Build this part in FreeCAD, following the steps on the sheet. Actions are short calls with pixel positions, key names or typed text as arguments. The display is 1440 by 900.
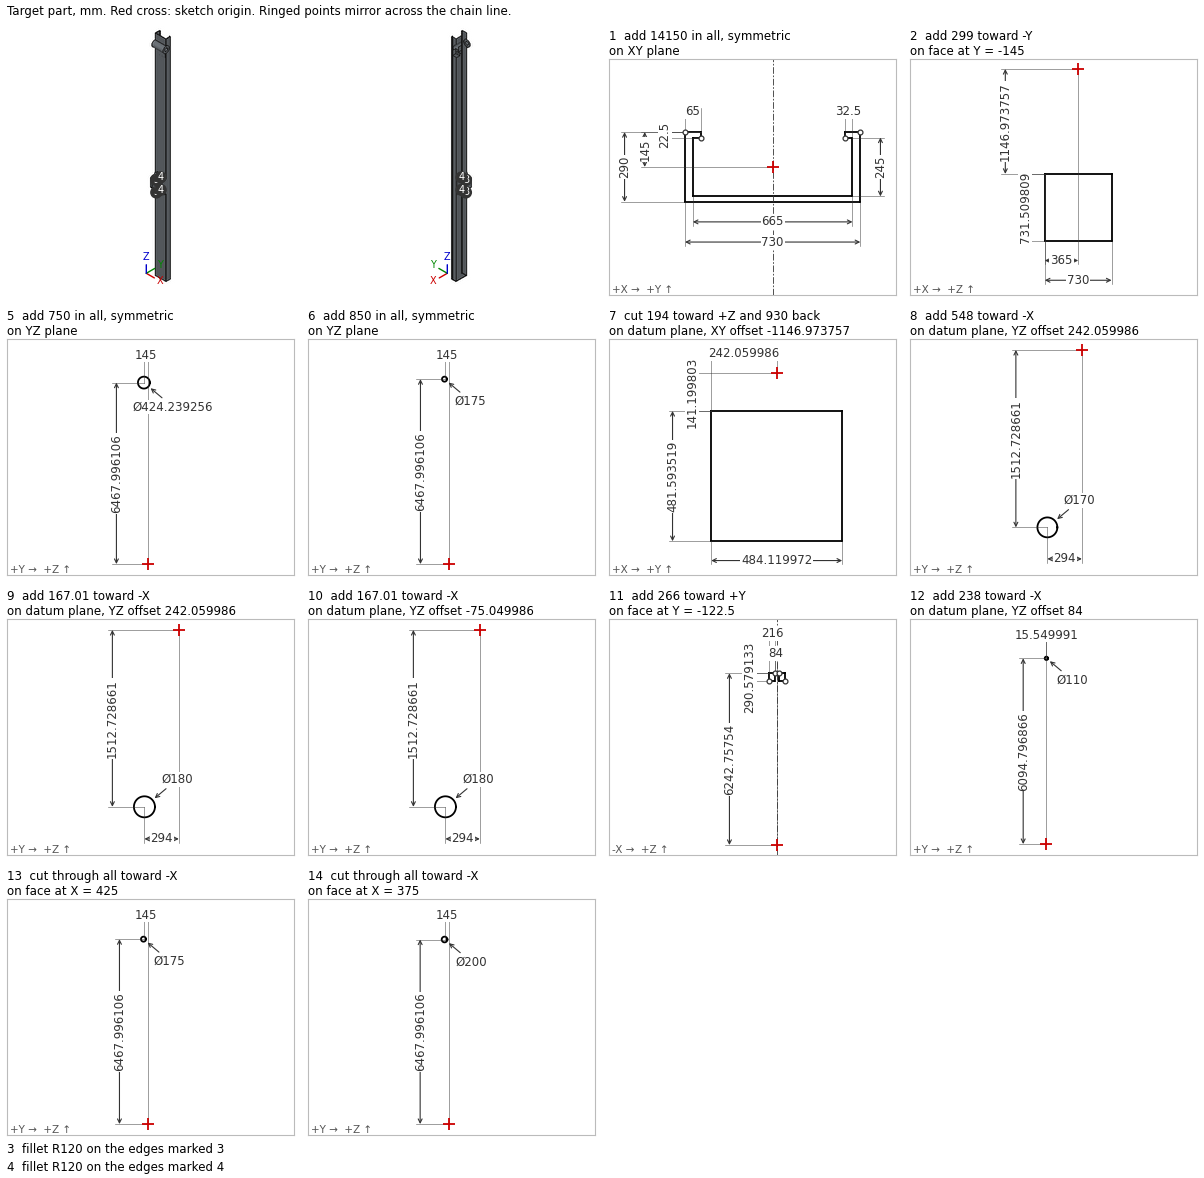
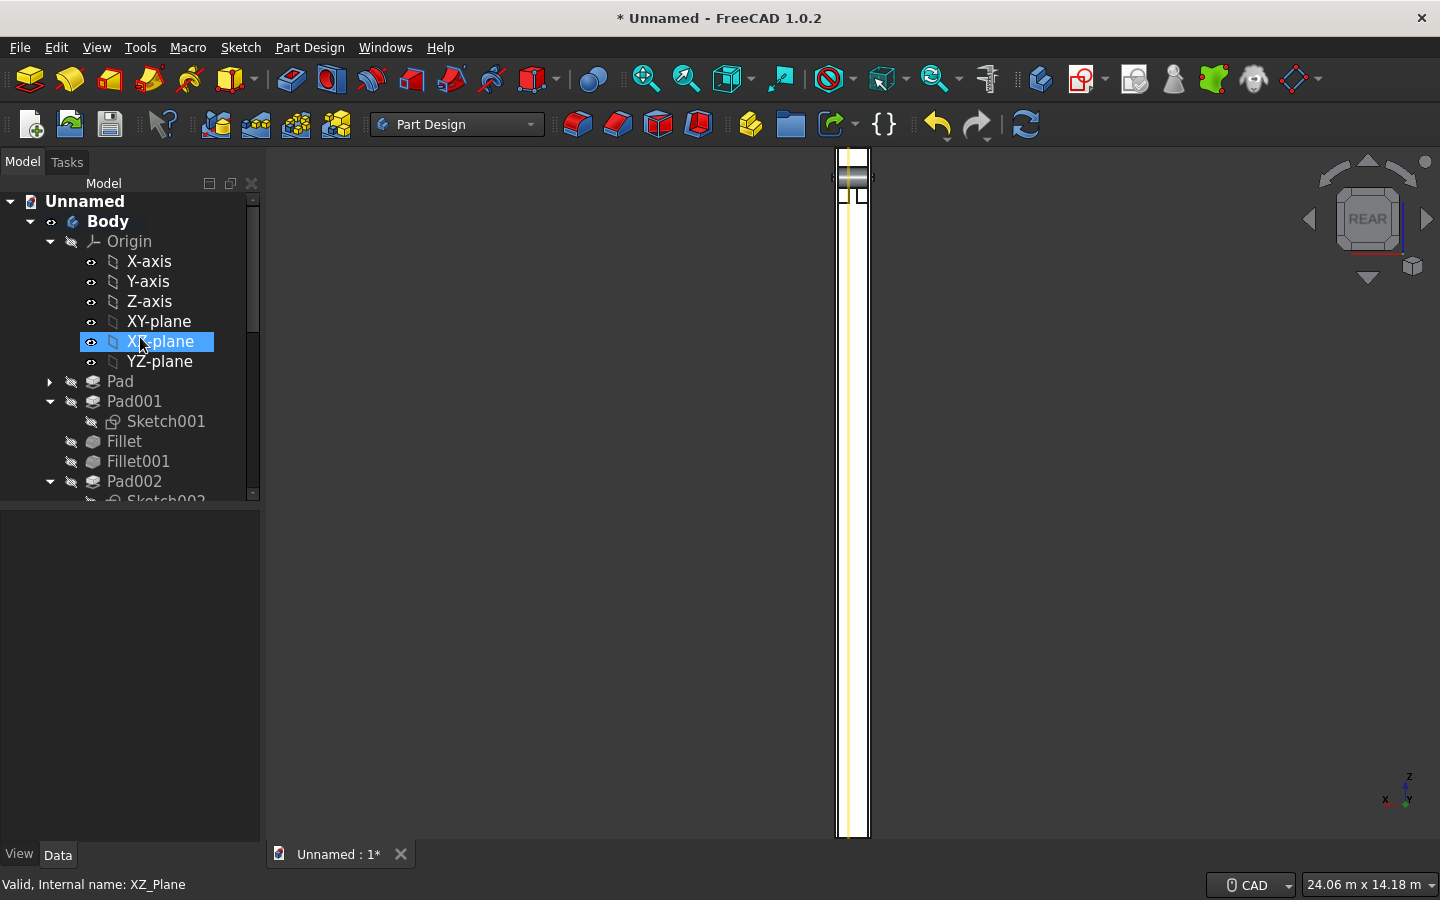
scroll(100, 337, down, 6)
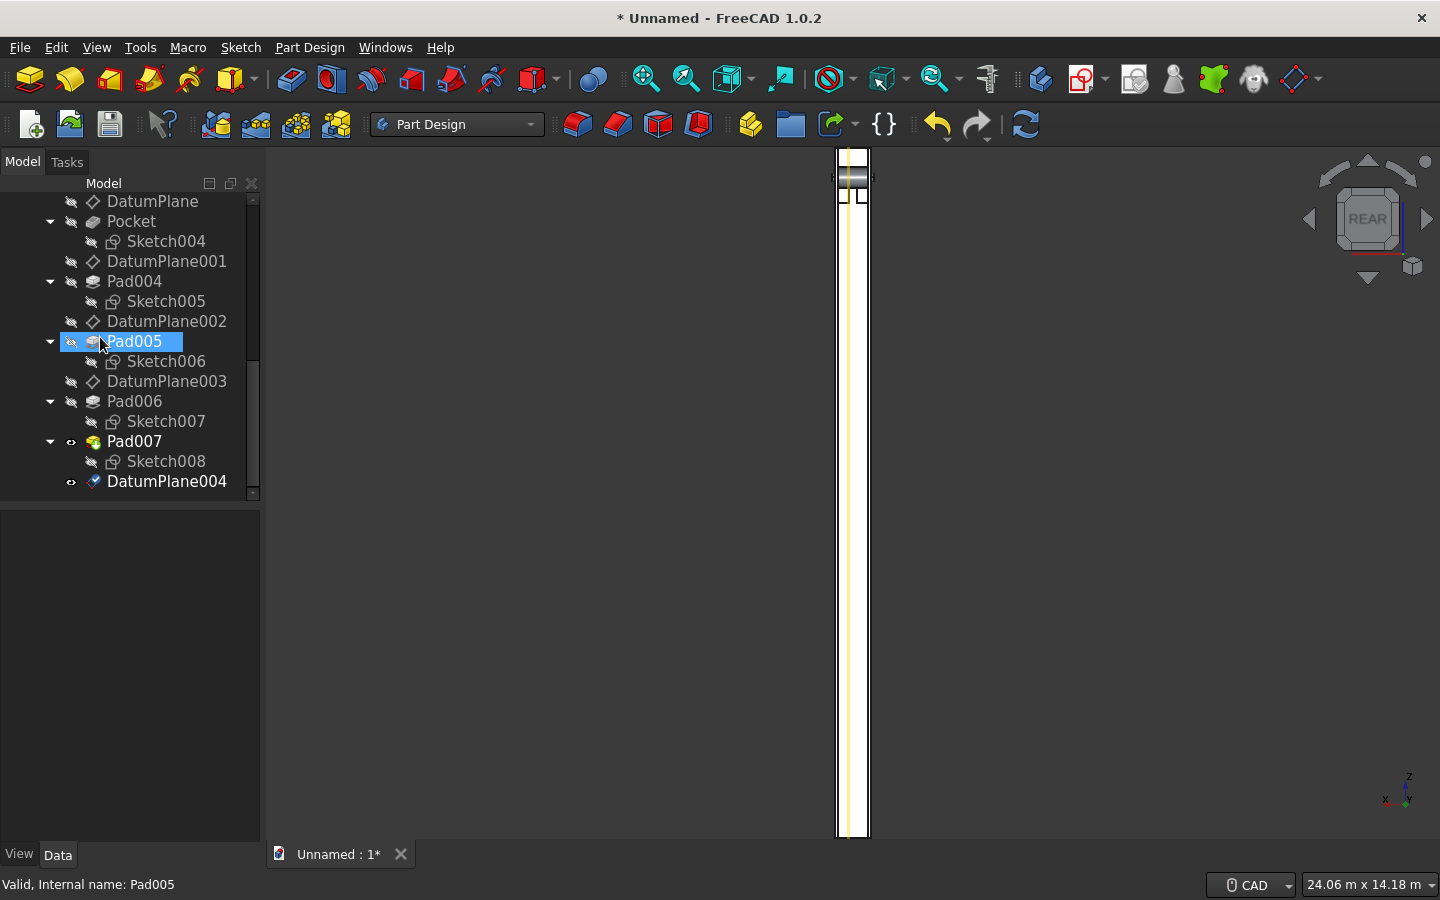
click(116, 482)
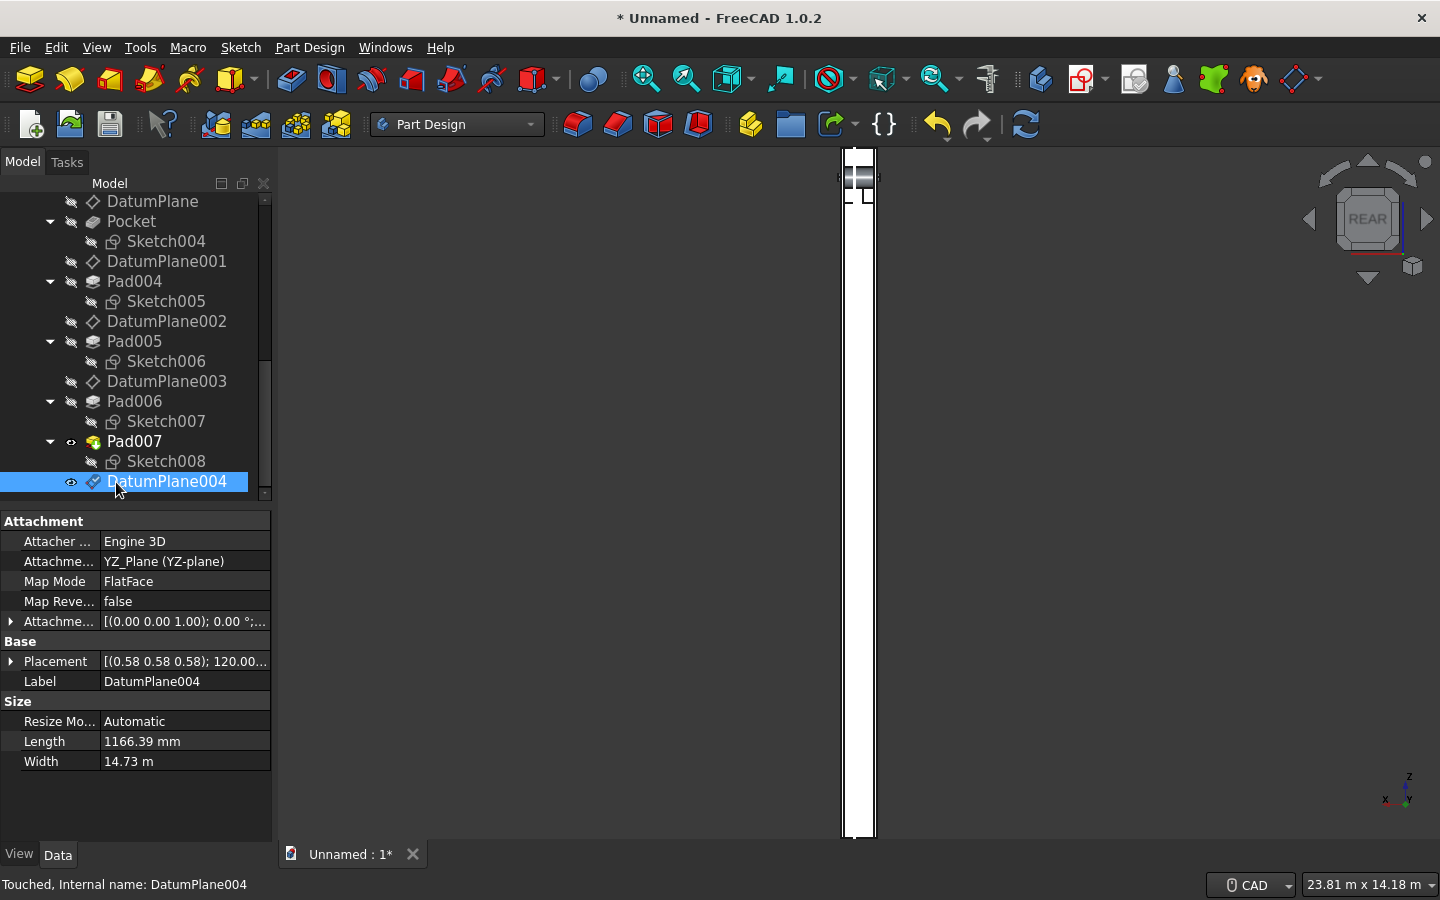
click(1082, 80)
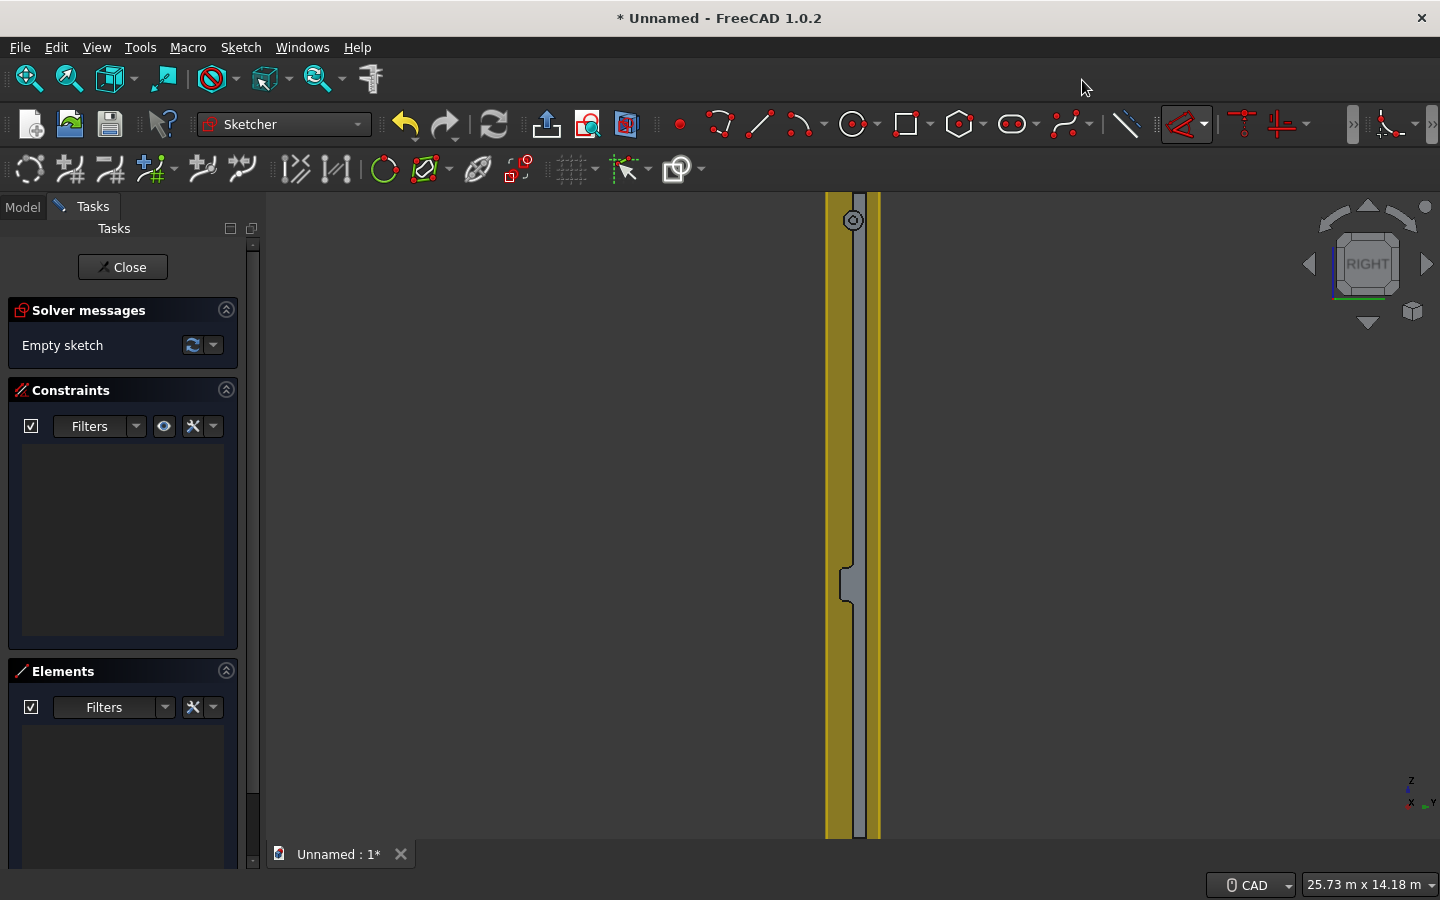
click(628, 124)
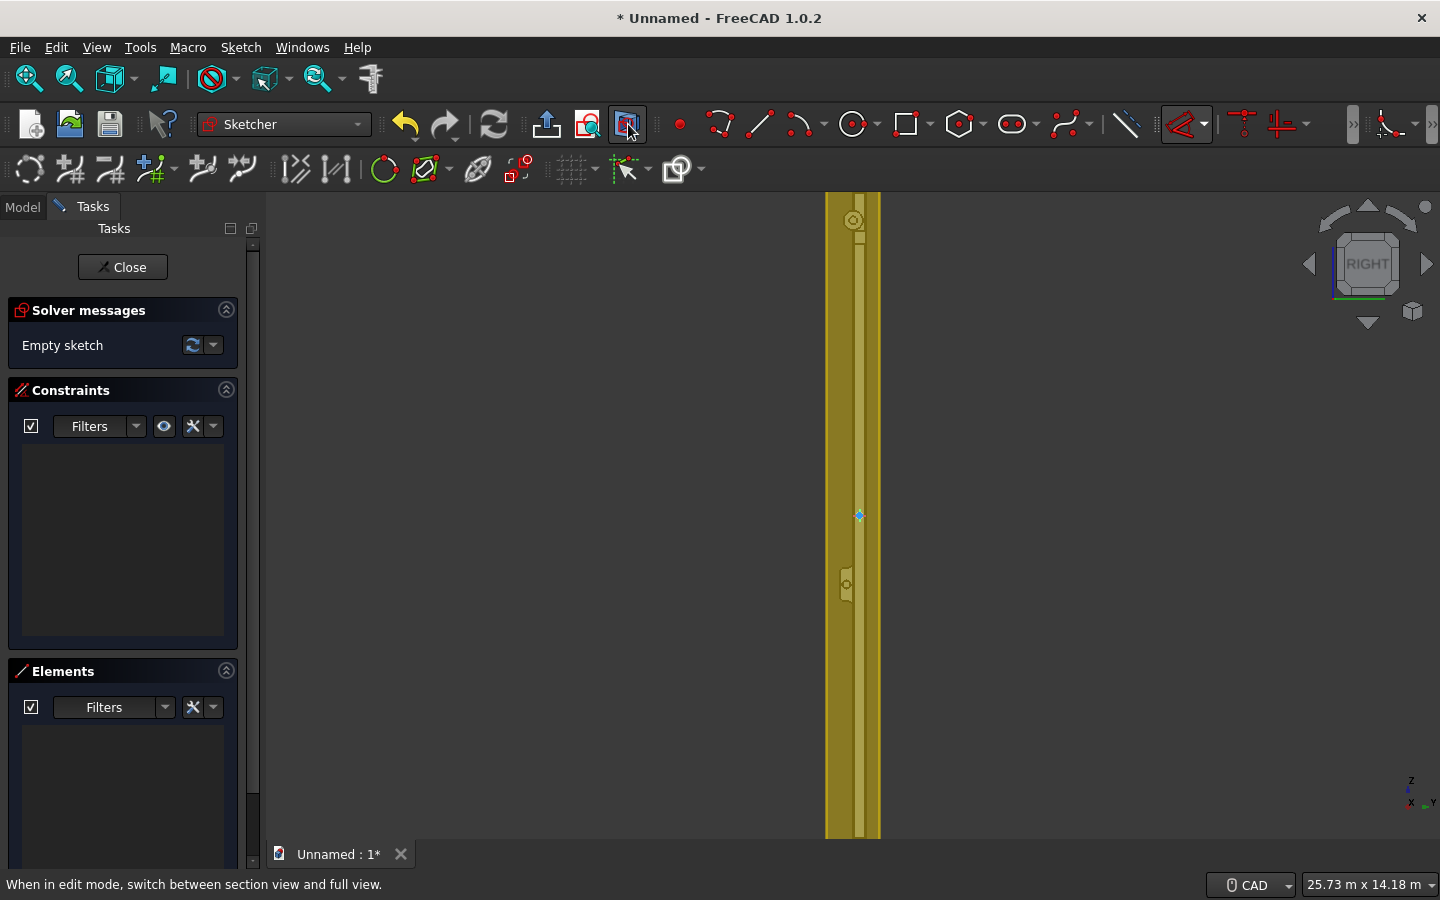
scroll(865, 223, up, 15)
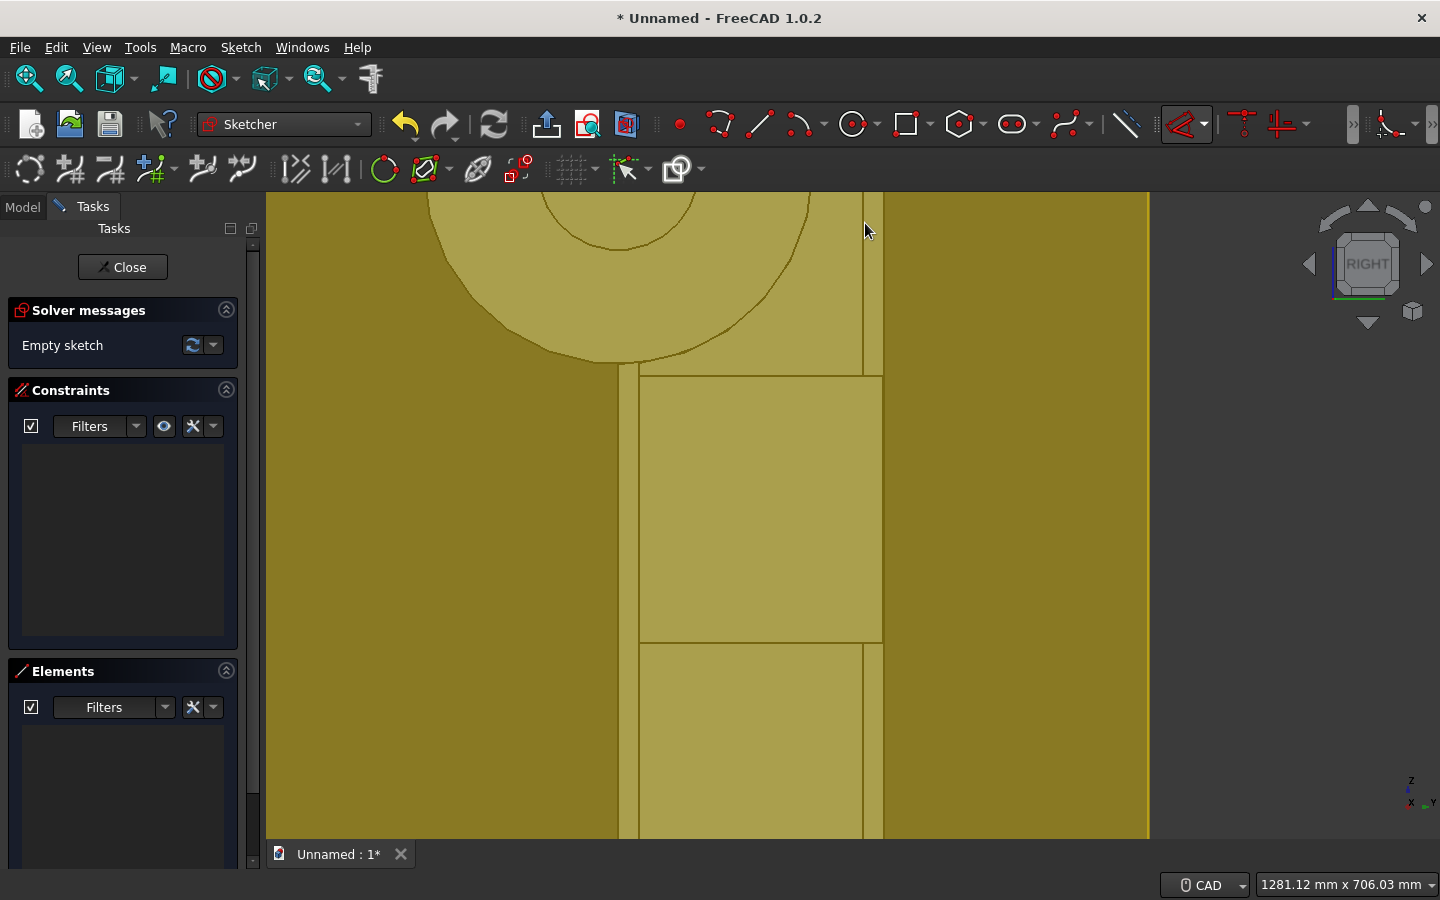
scroll(759, 511, up, 7)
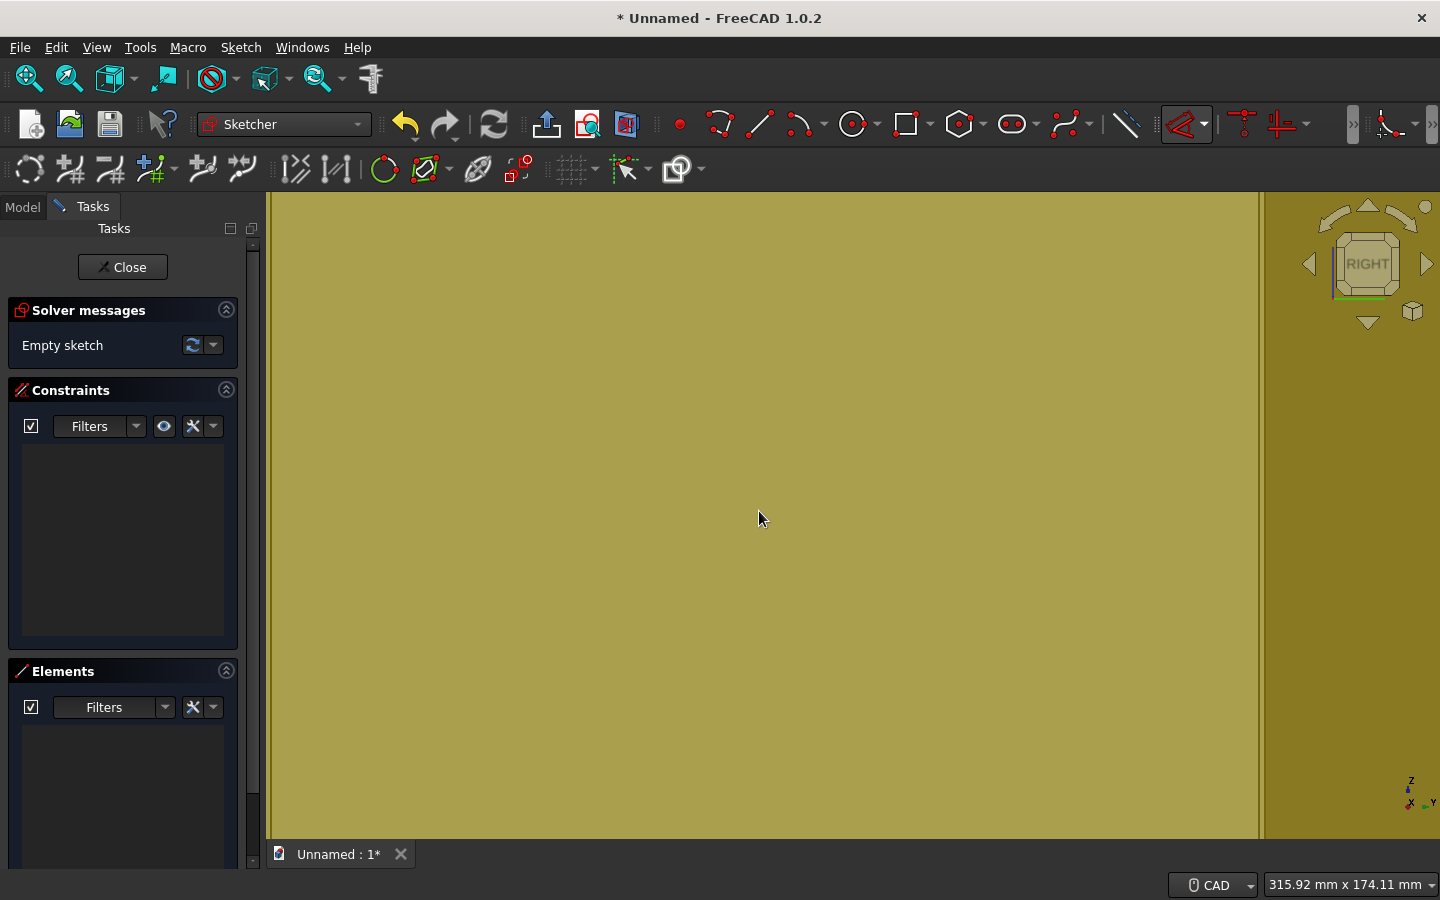
key(g)
key(c)